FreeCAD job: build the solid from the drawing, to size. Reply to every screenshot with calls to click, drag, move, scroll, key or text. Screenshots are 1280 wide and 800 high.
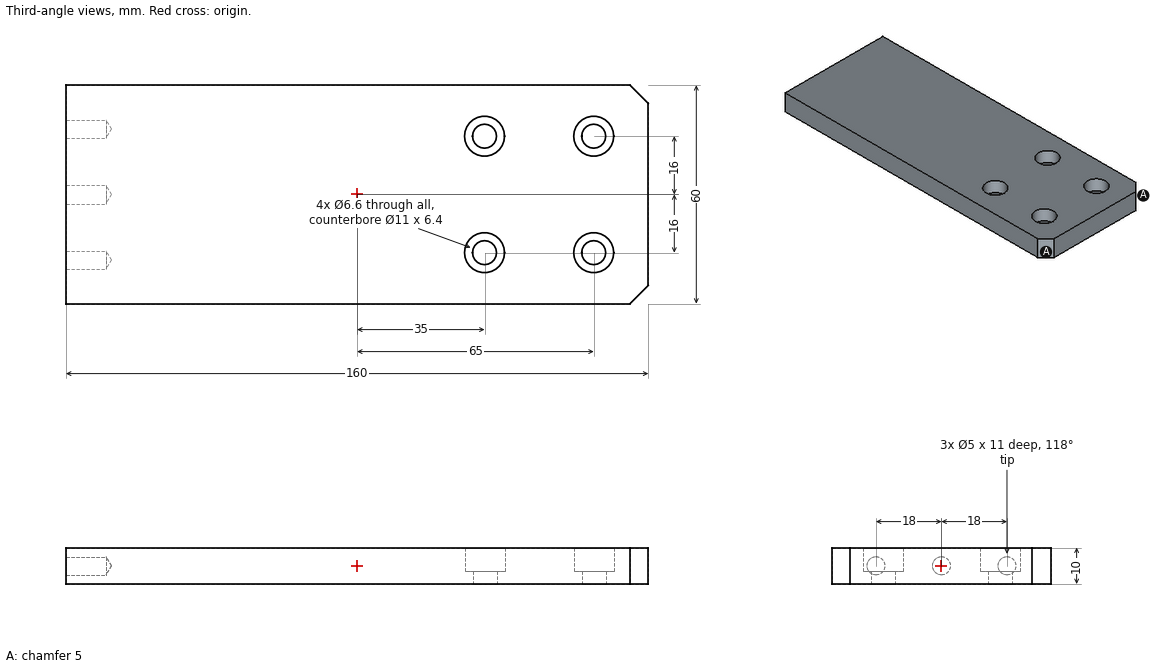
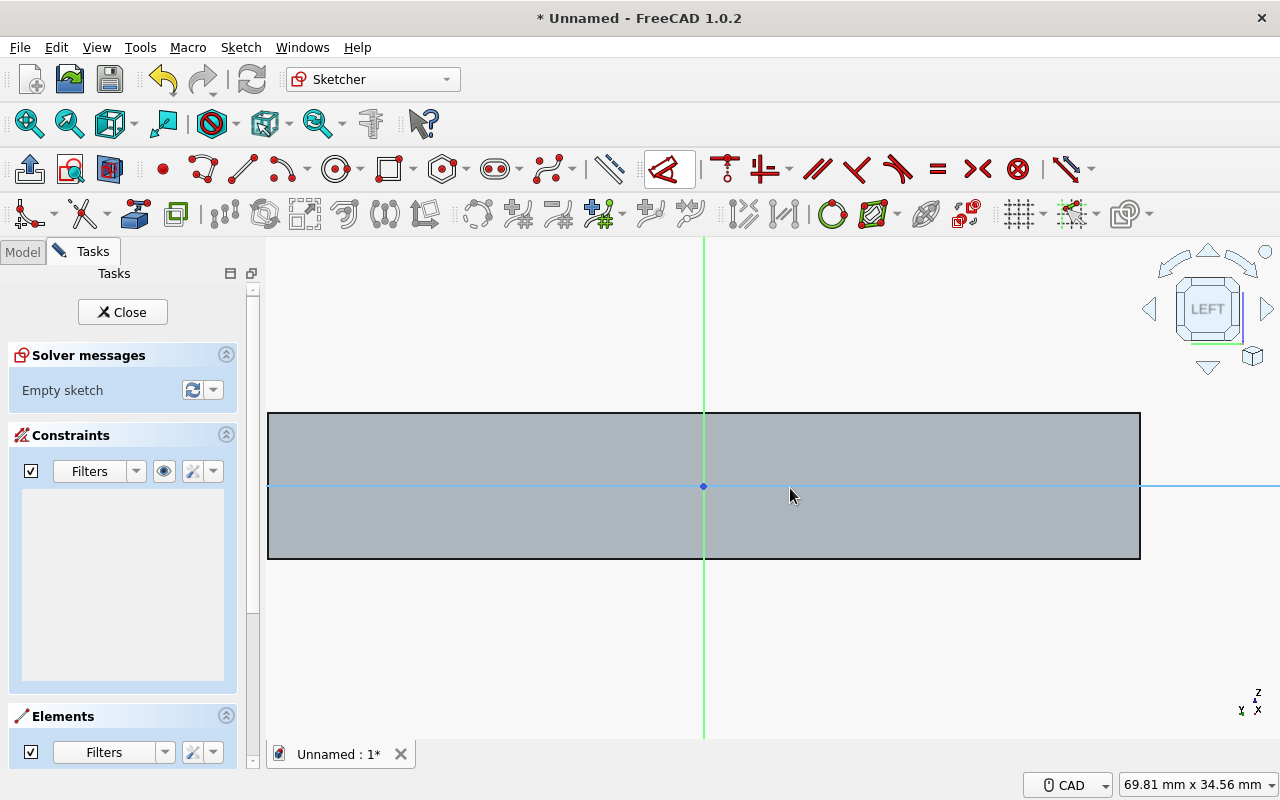
click(336, 170)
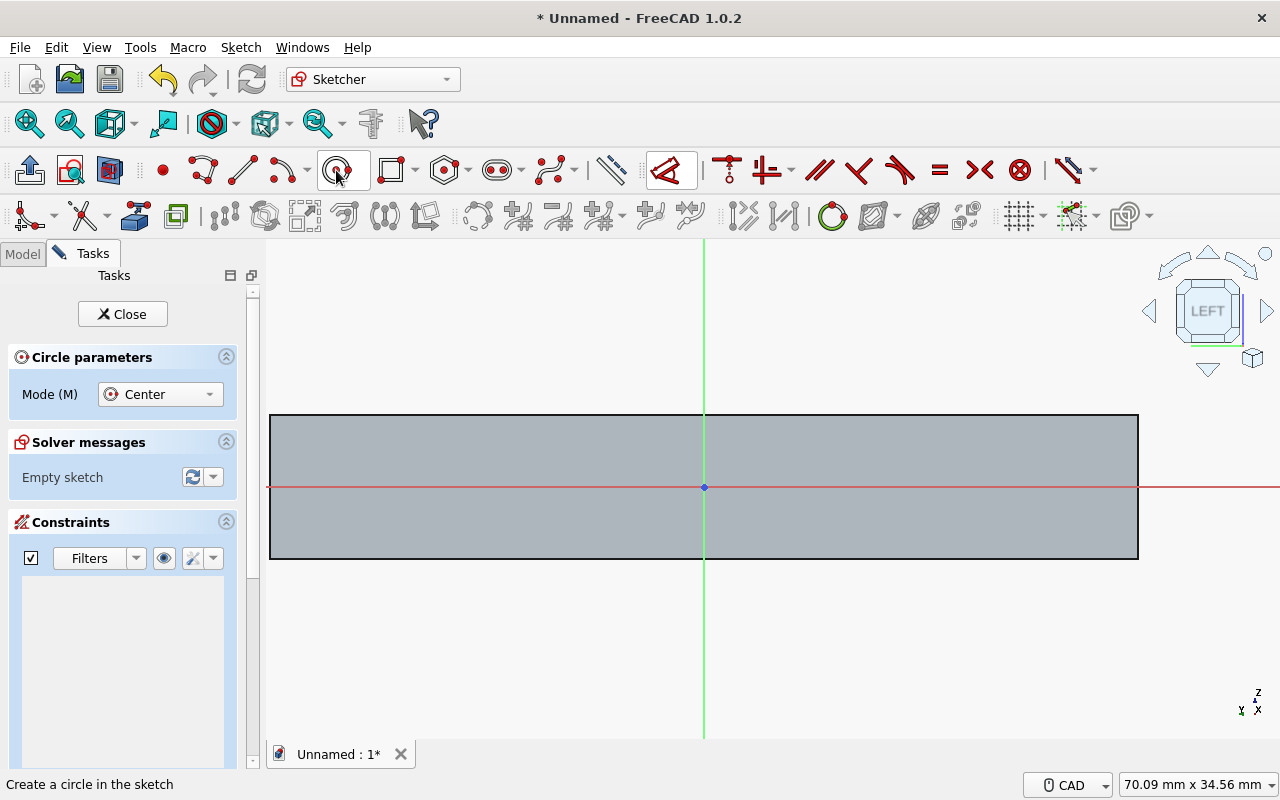
click(444, 487)
move(469, 461)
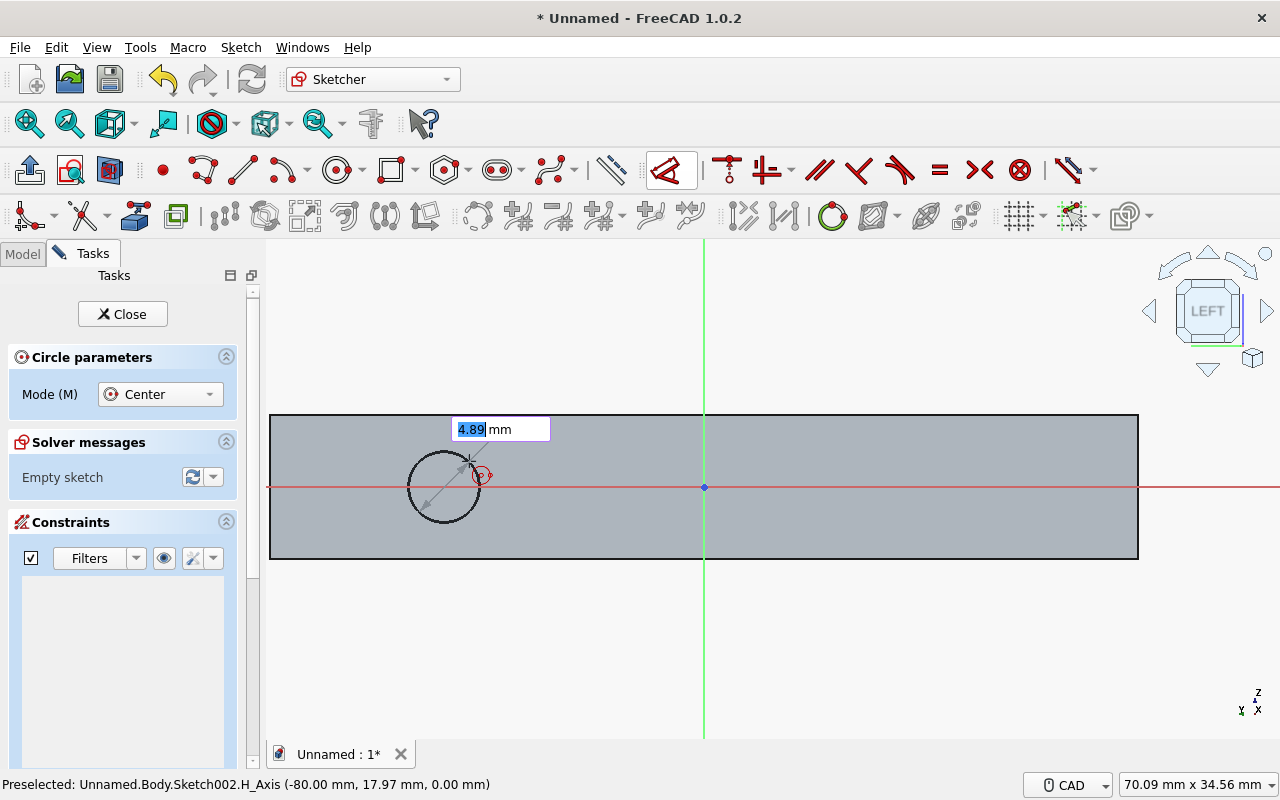
text(5)
key(Return)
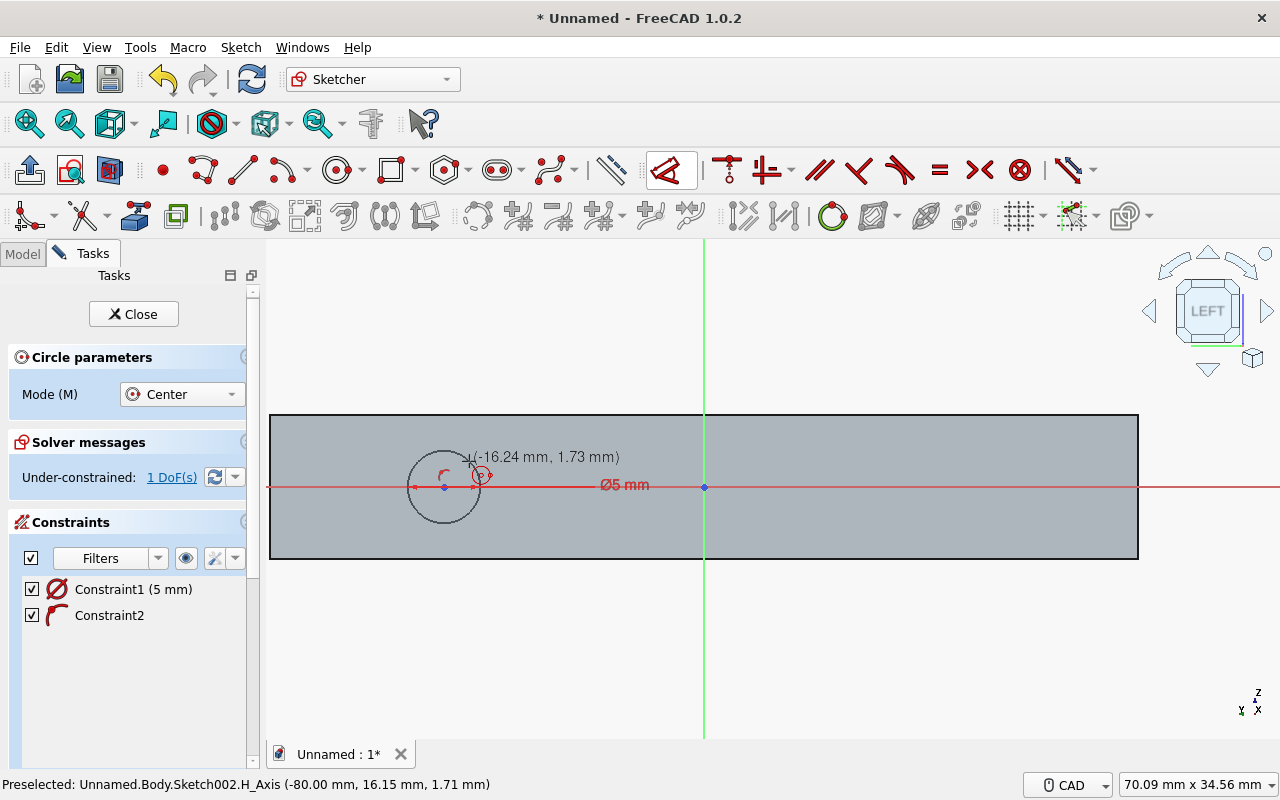
click(704, 487)
move(730, 461)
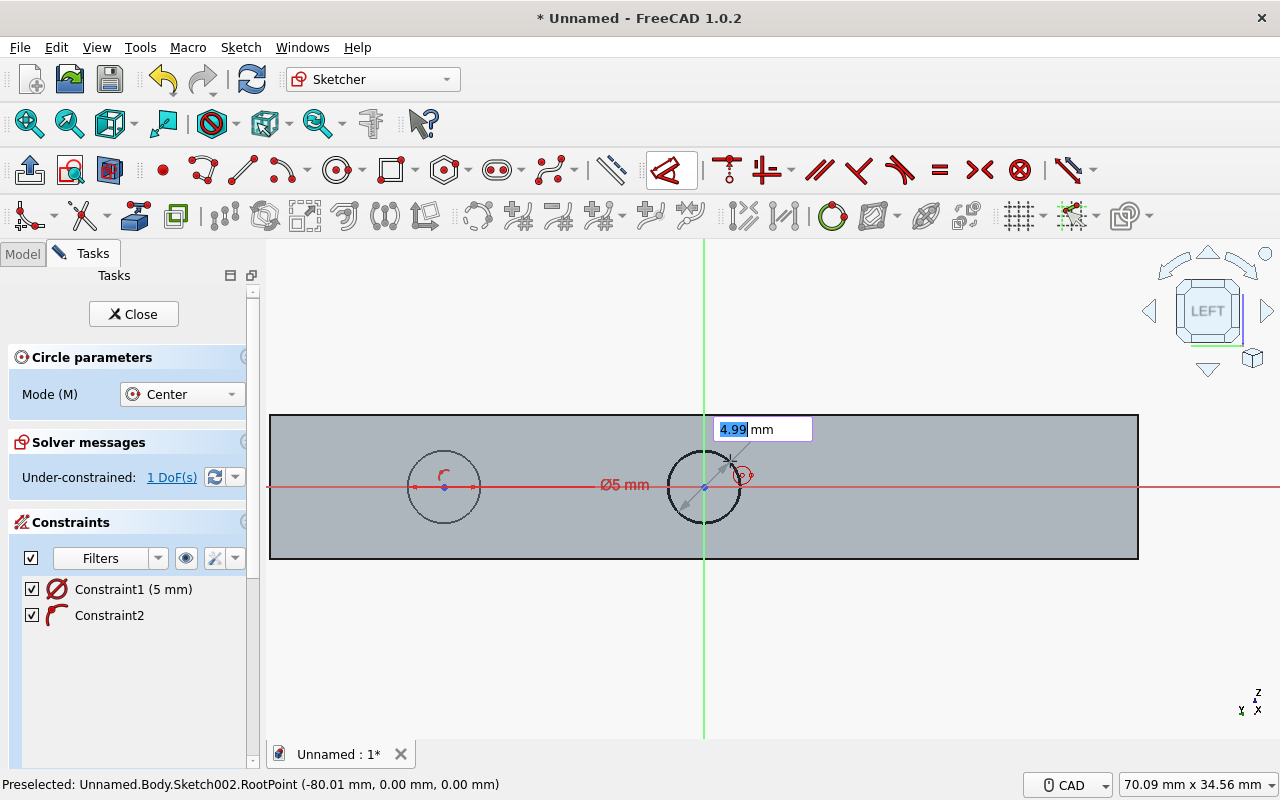
text(5)
key(Return)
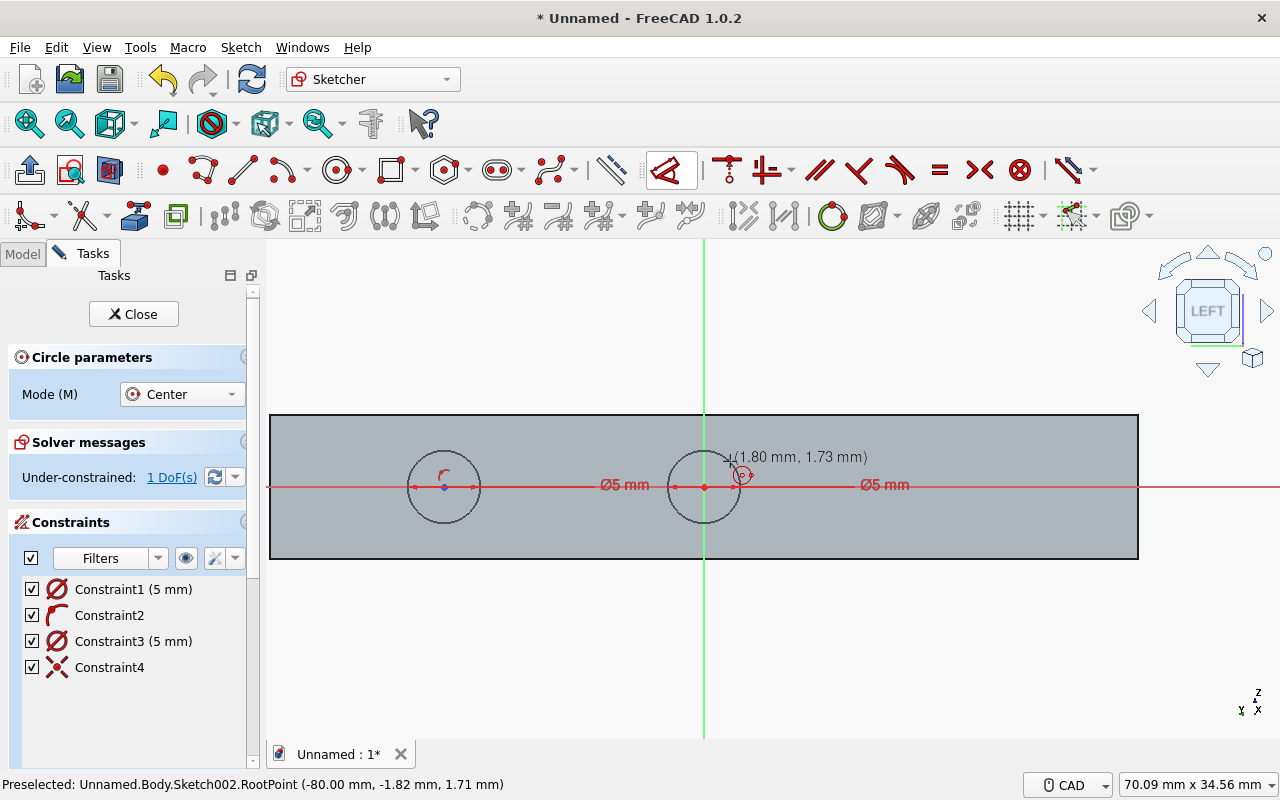
click(964, 487)
move(990, 461)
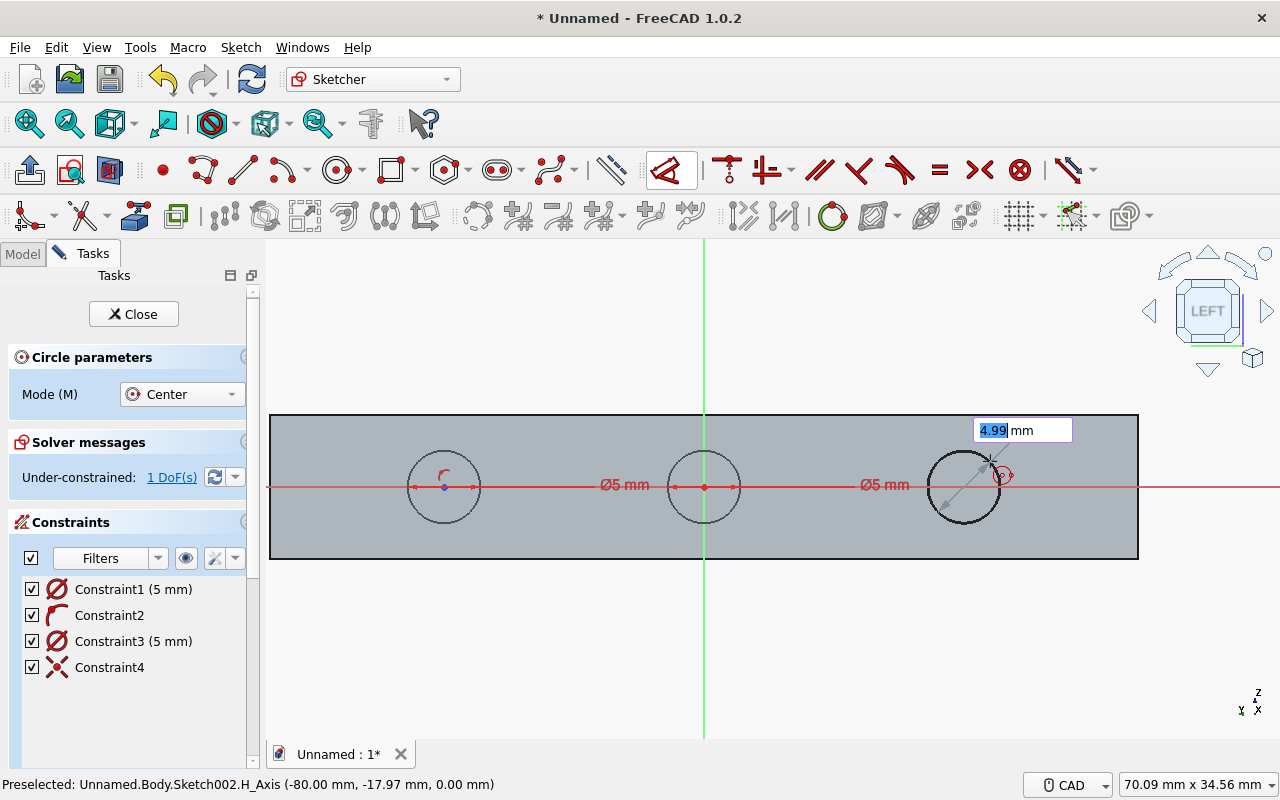
text(5)
key(Return)
key(Escape)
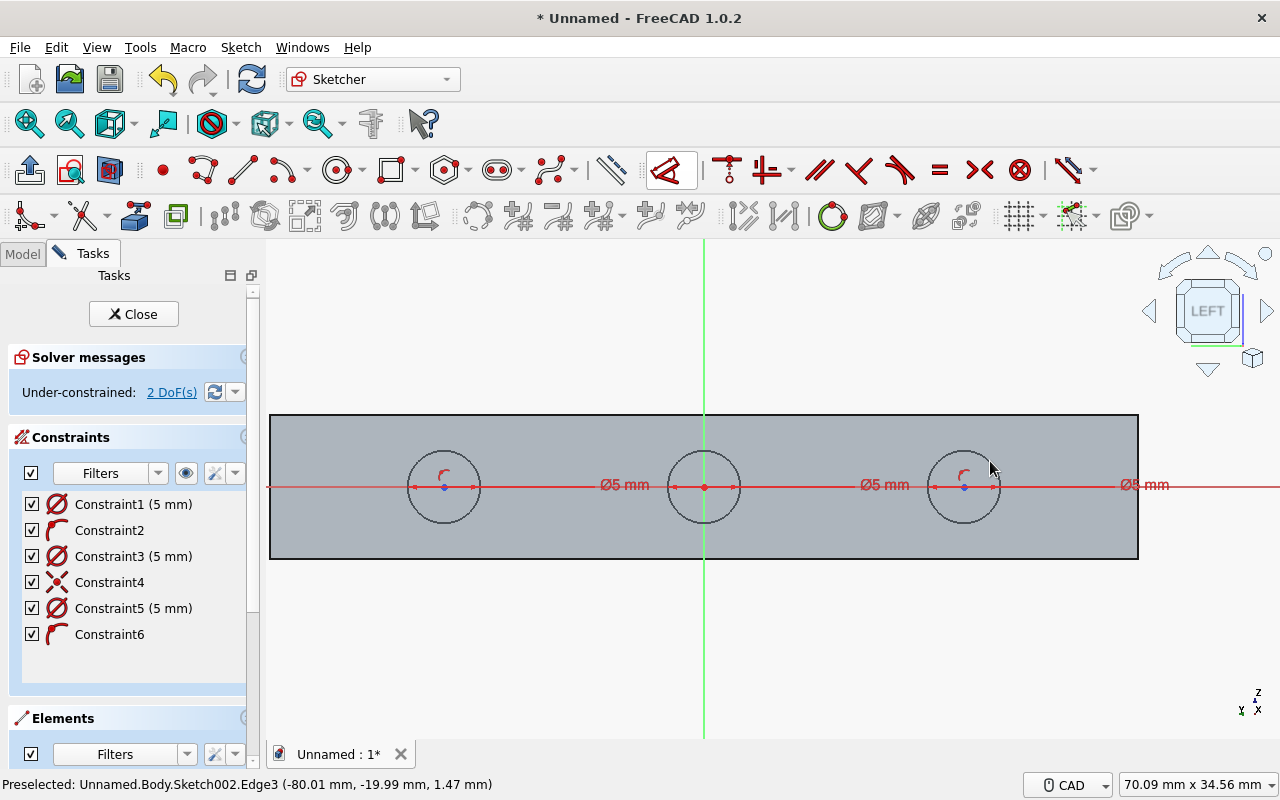
click(444, 487)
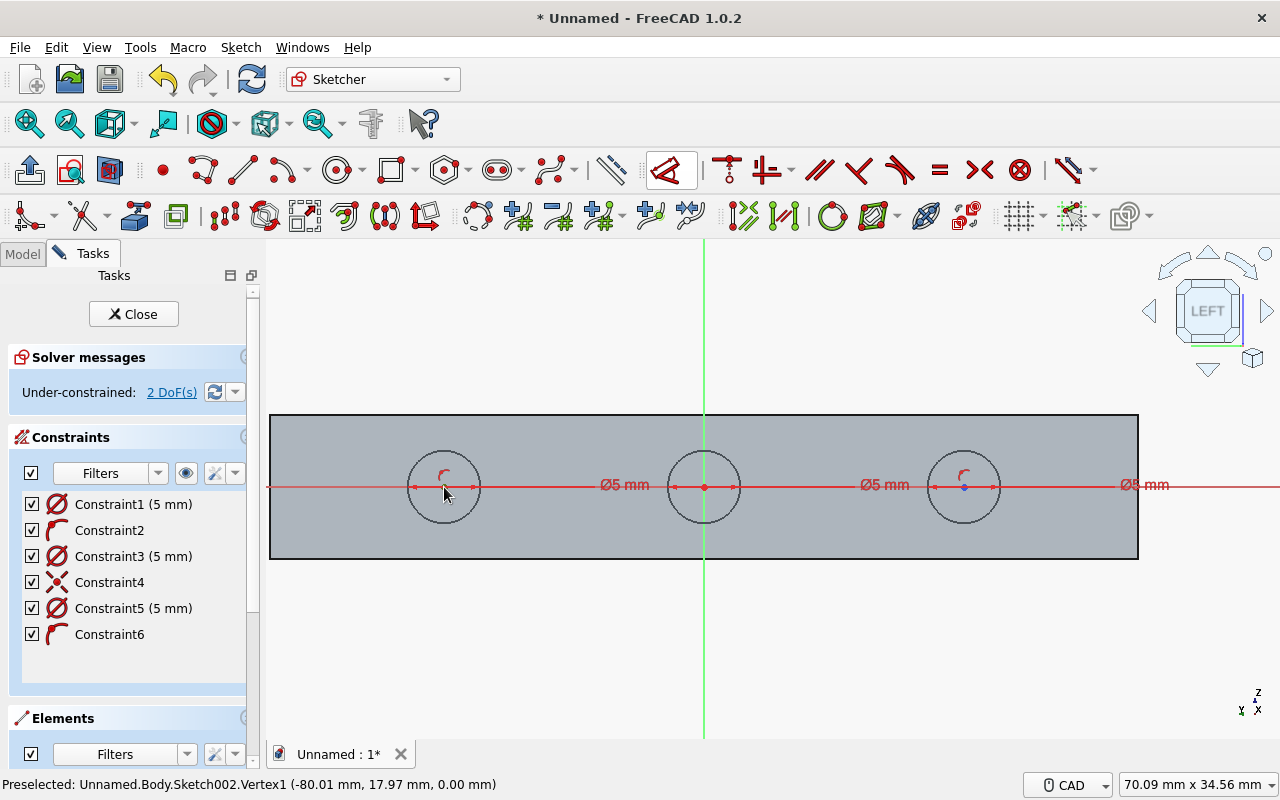
key(l)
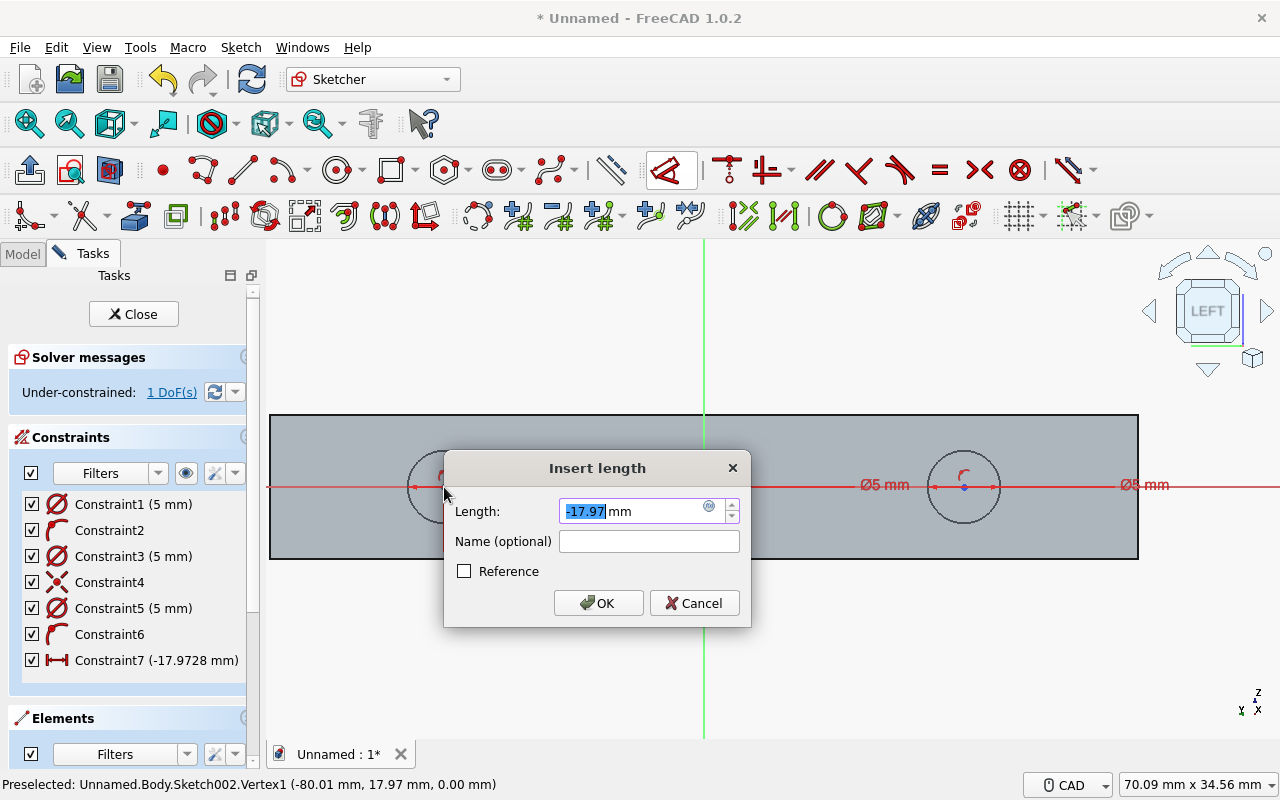
text(-18)
key(Return)